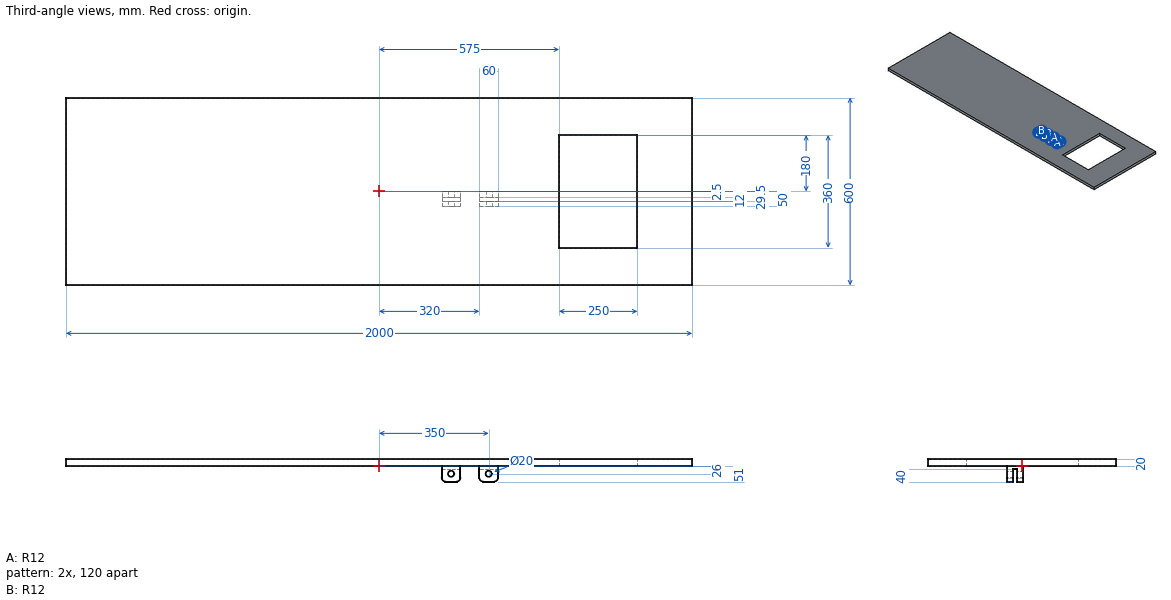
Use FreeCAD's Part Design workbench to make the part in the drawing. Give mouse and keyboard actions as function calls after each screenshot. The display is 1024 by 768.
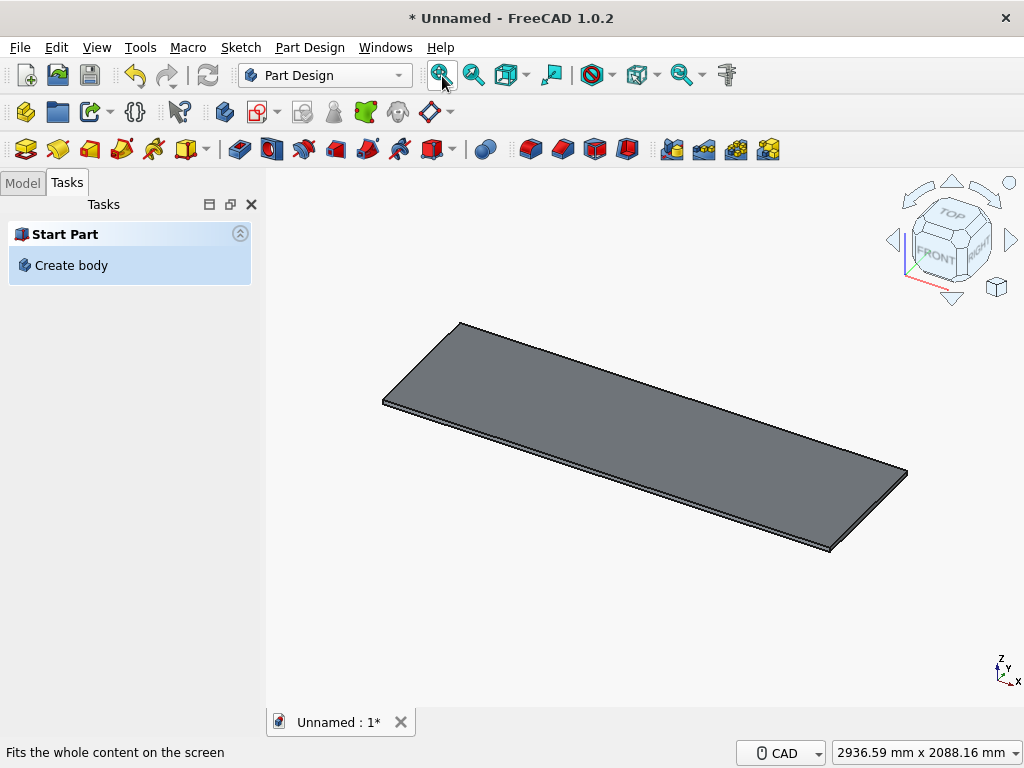
click(258, 112)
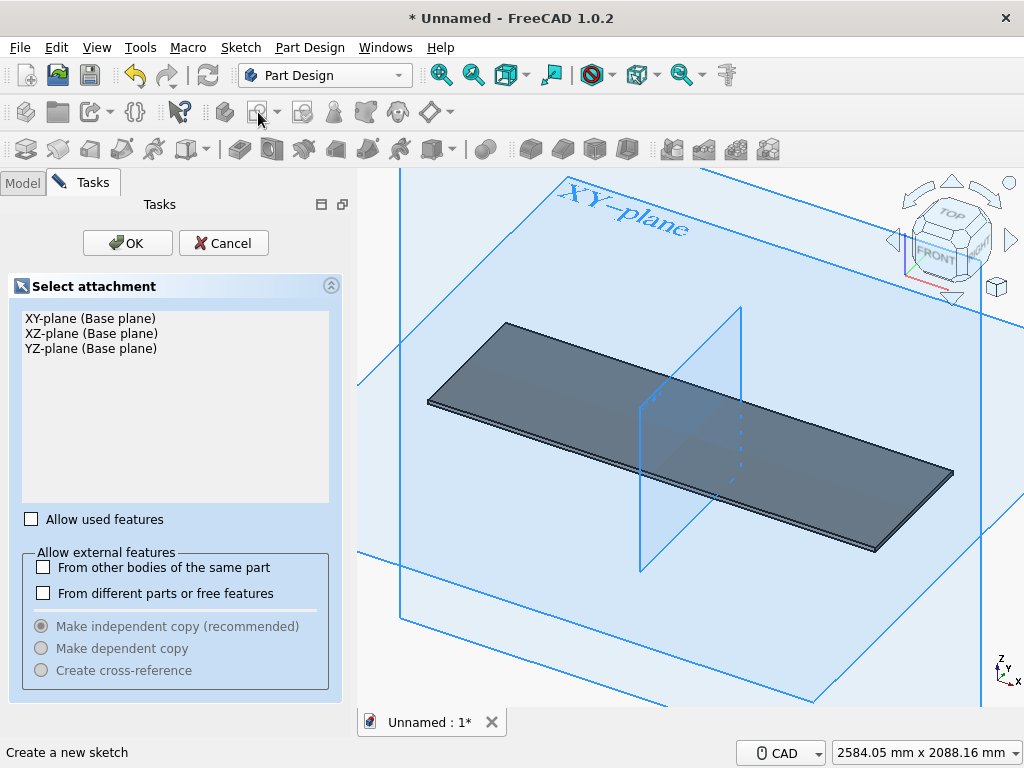
click(82, 318)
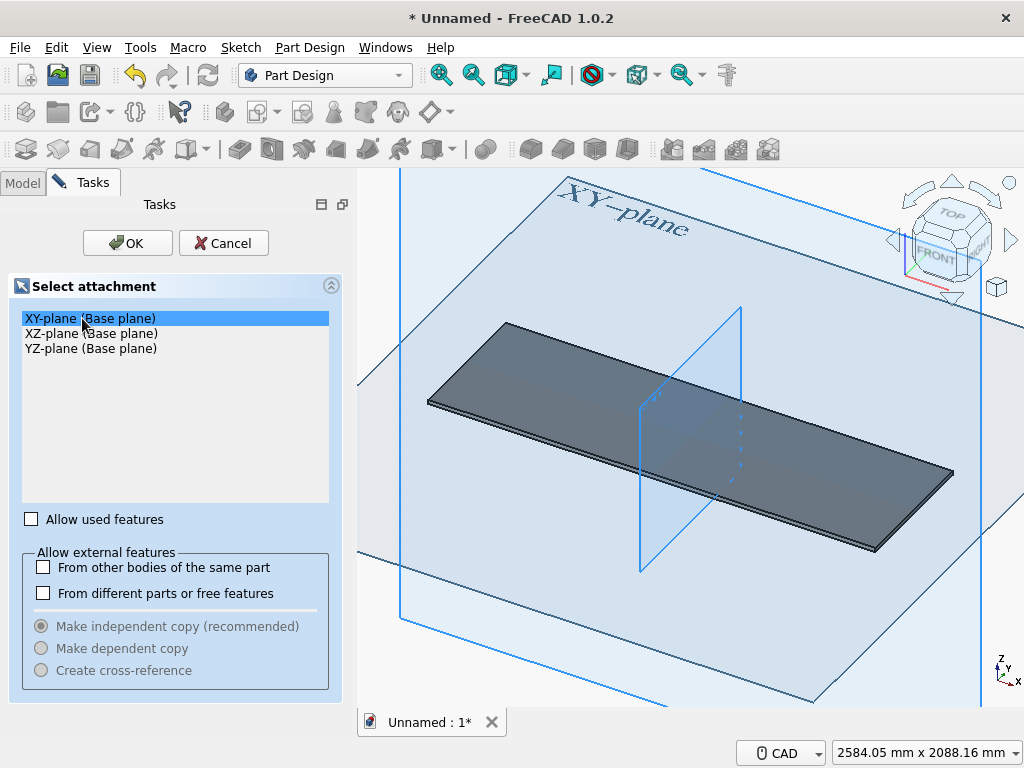
click(128, 243)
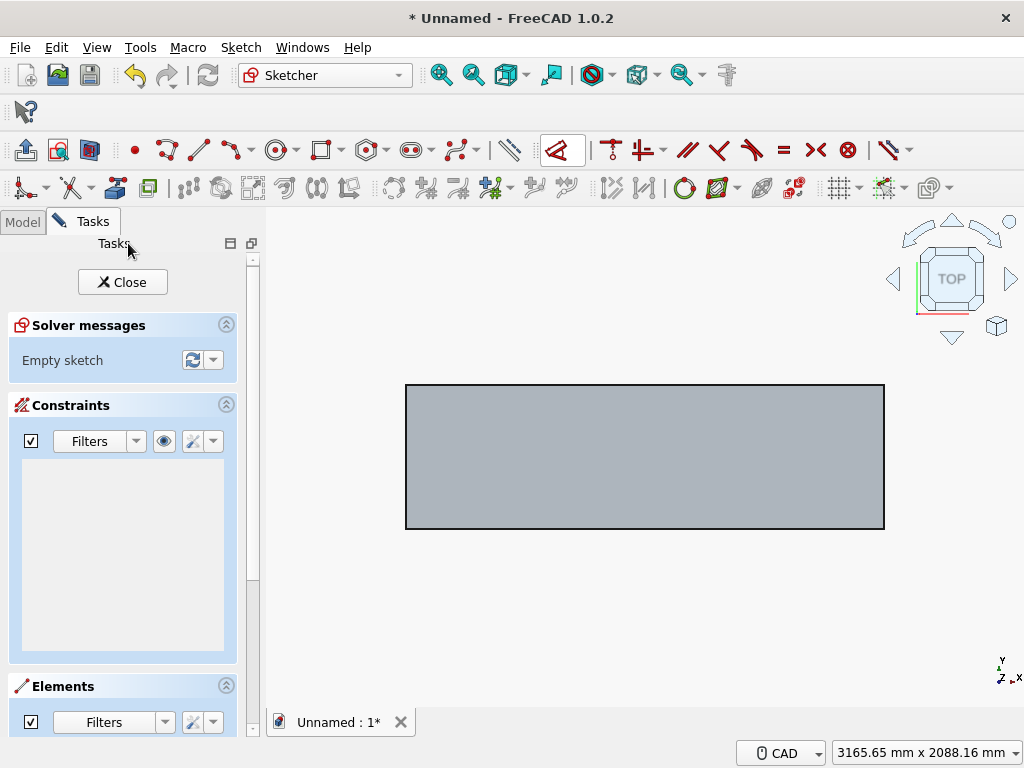
key(q)
key(s)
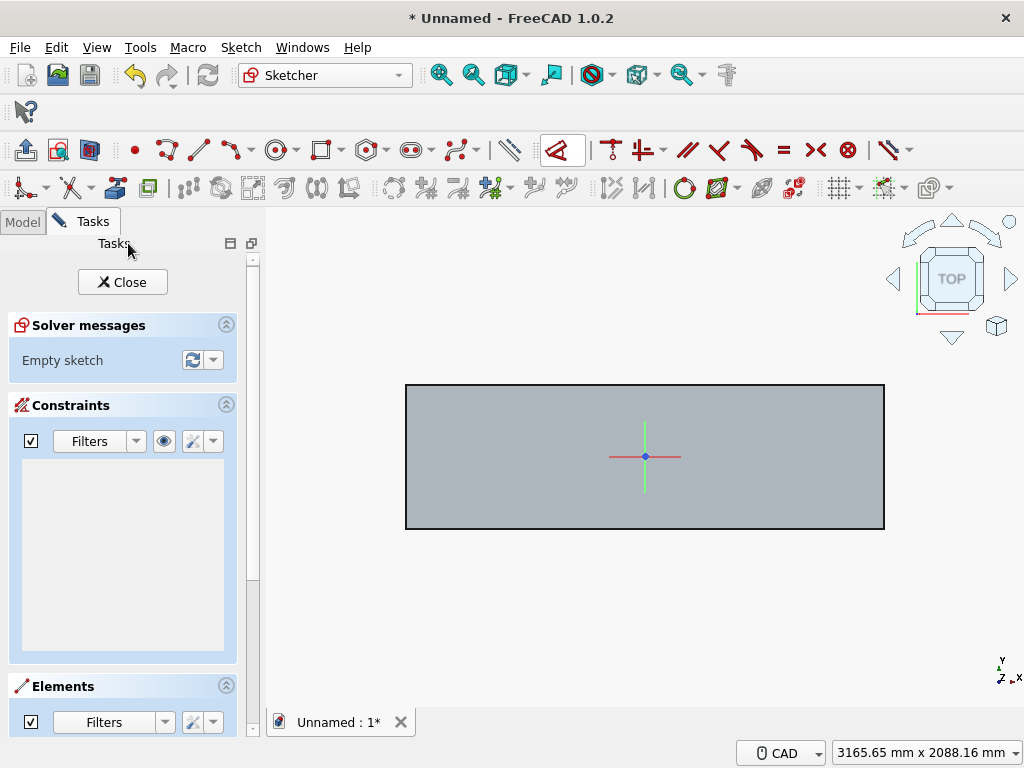
scroll(859, 457, up, 4)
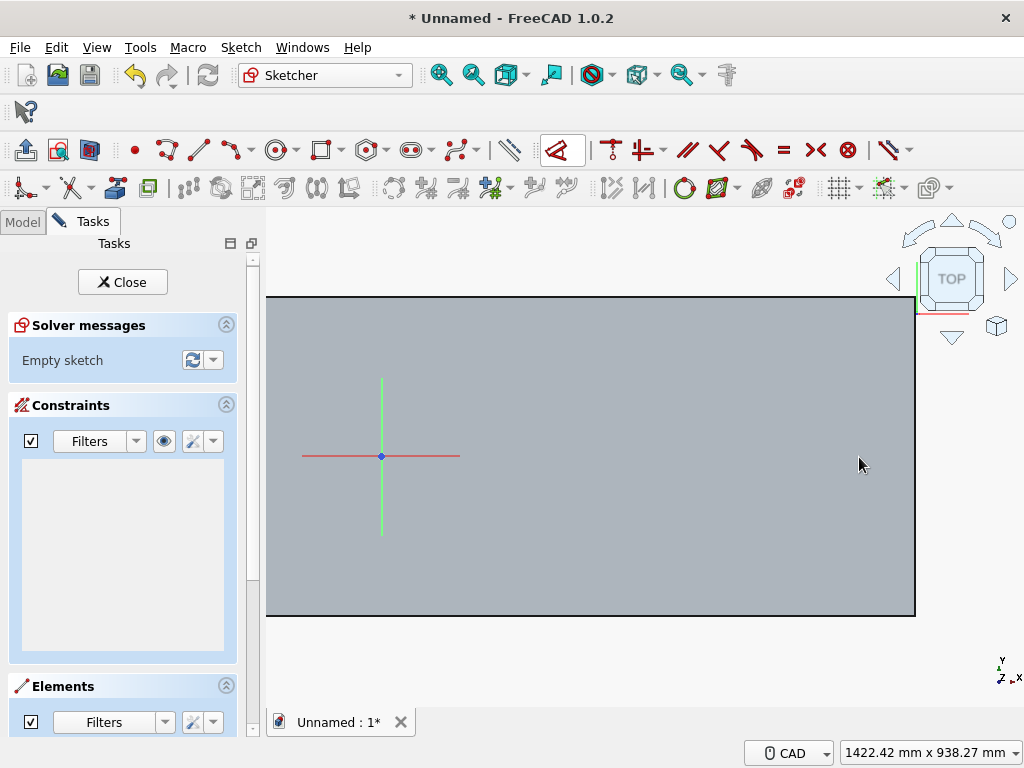
key(g)
key(r)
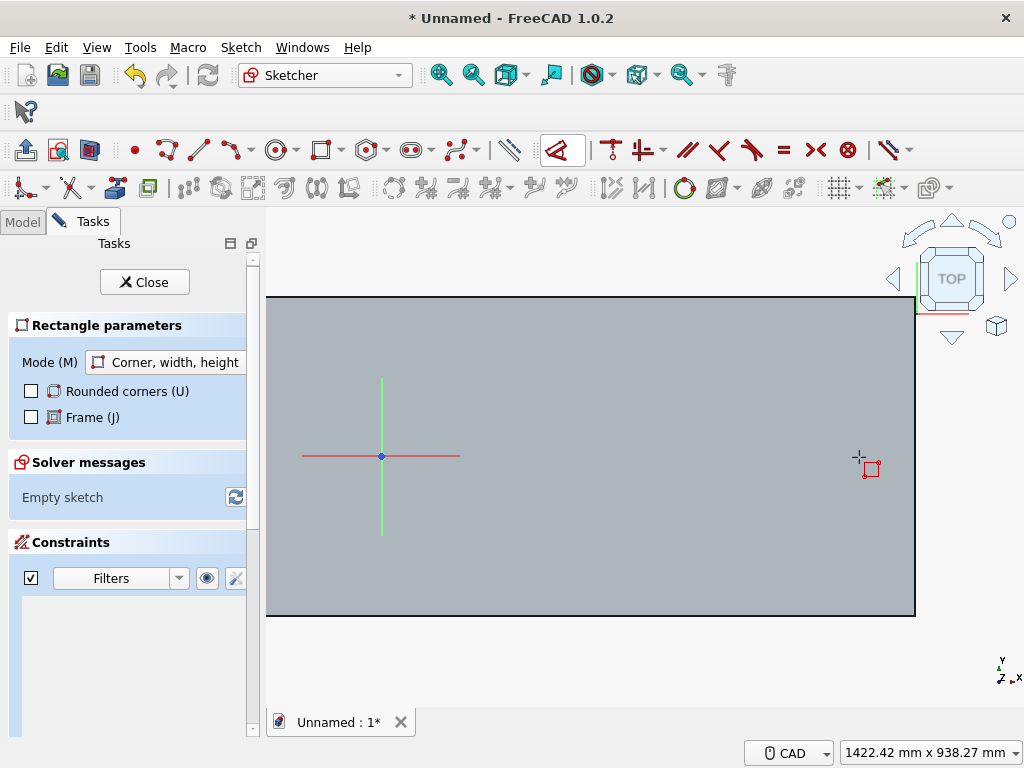
click(688, 360)
move(821, 552)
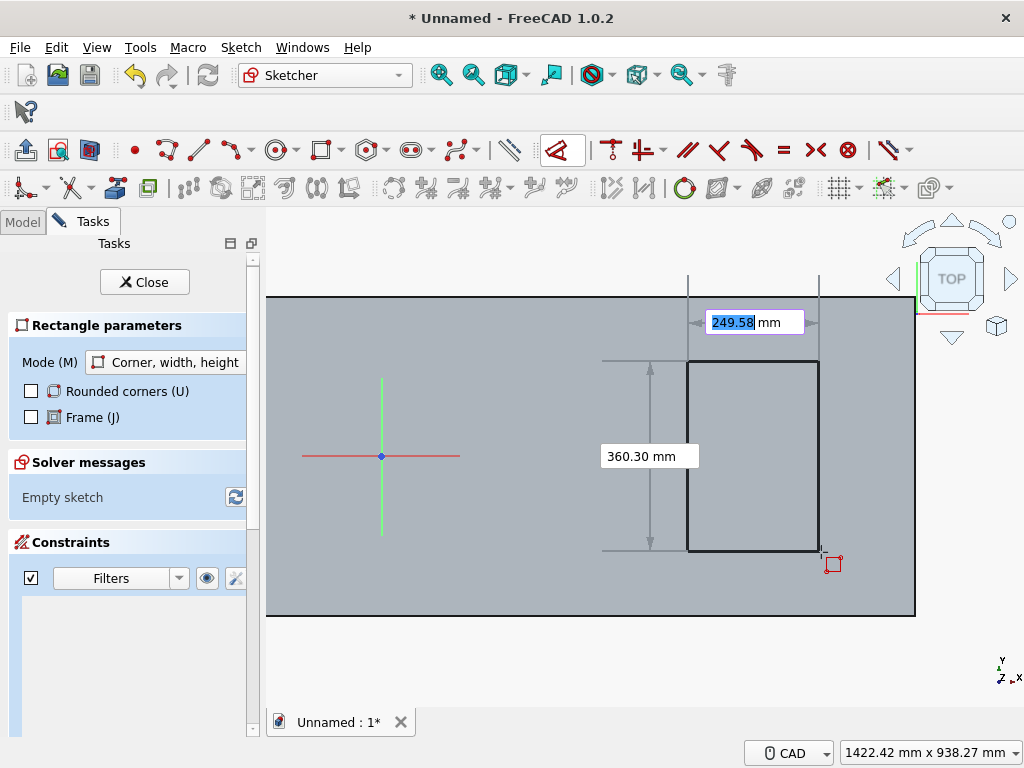
text(250)
key(Tab)
text(360)
key(Return)
key(Escape)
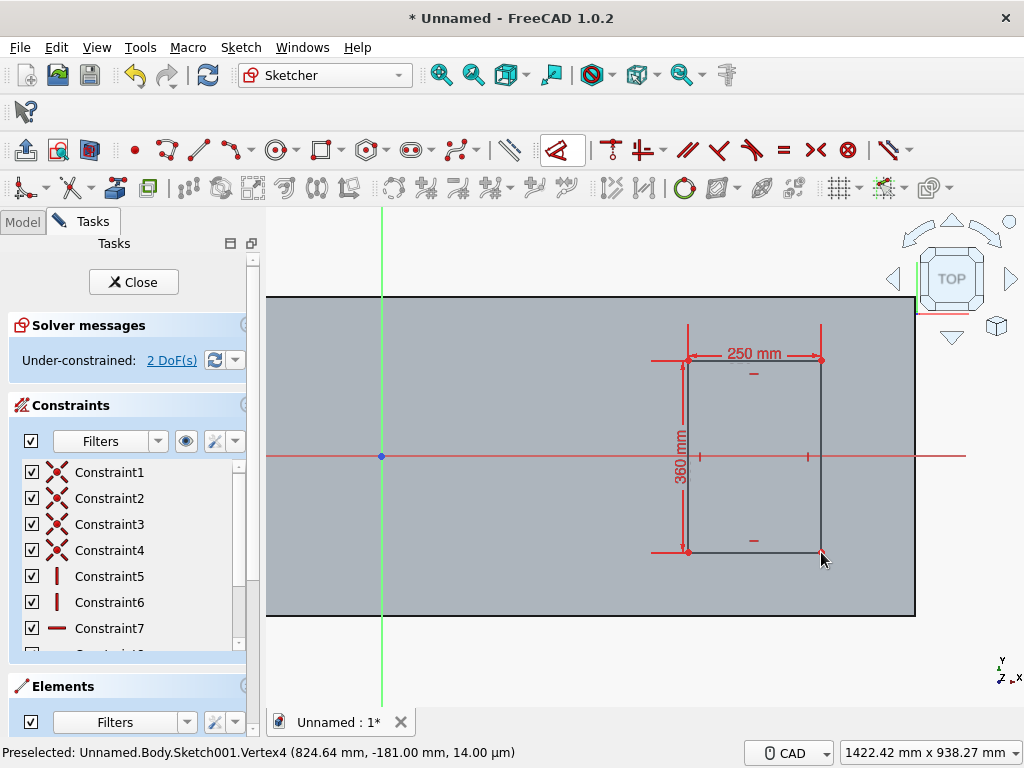
click(556, 150)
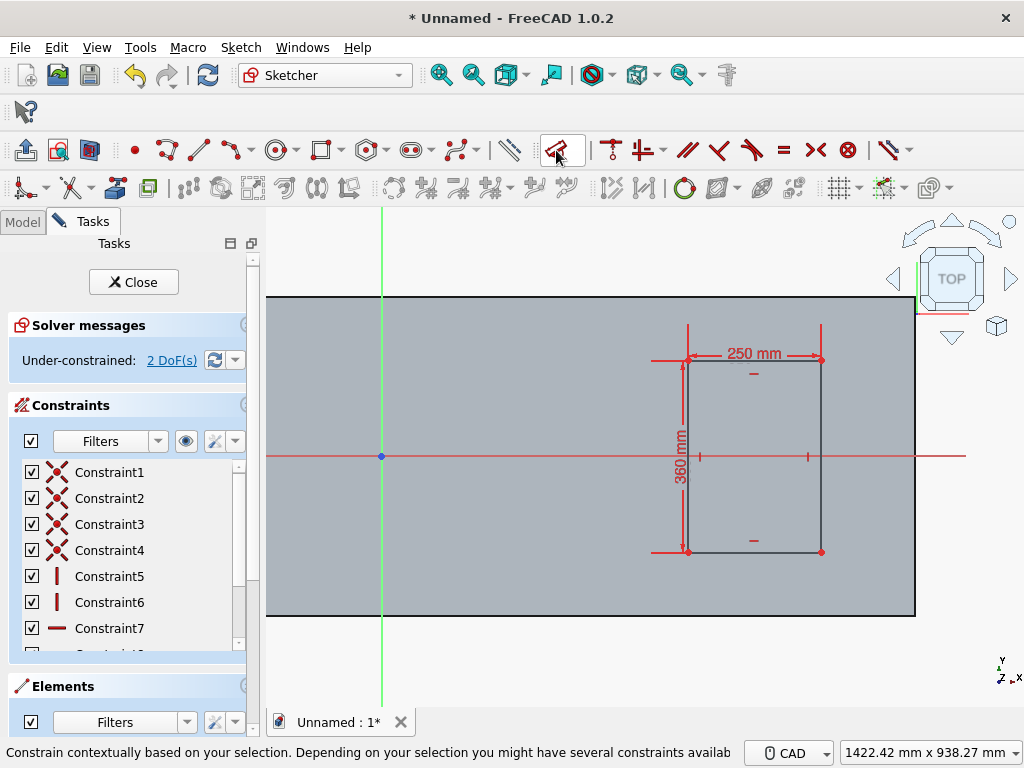
click(688, 361)
click(535, 327)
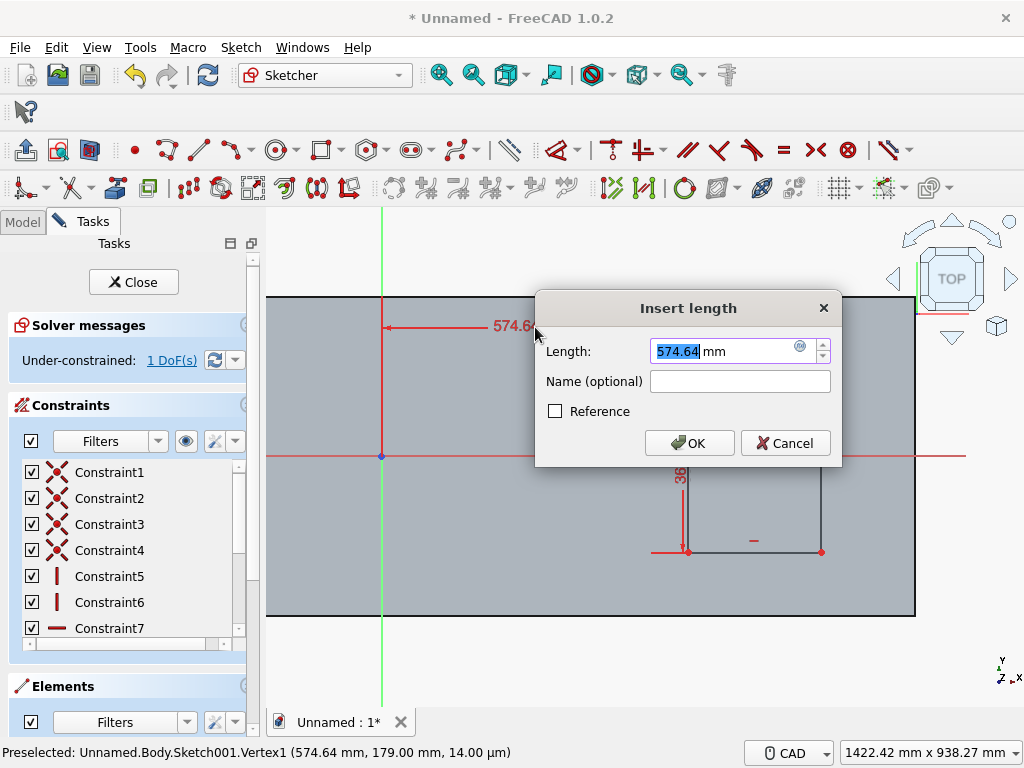
text(575)
key(Return)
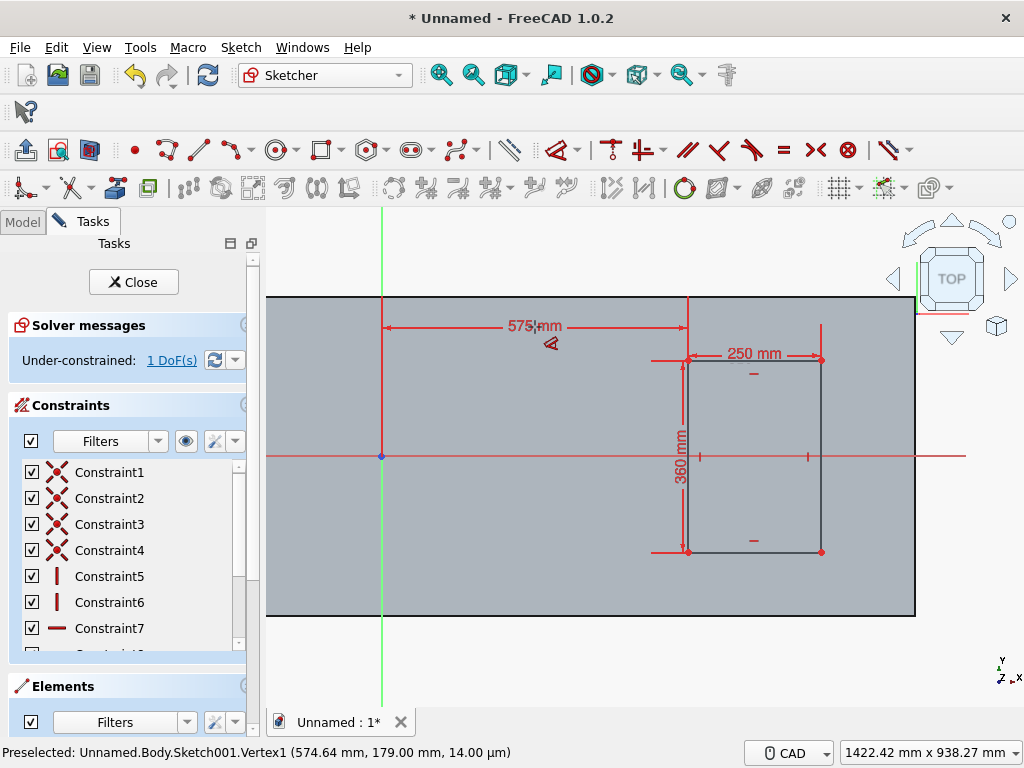
click(688, 361)
click(348, 409)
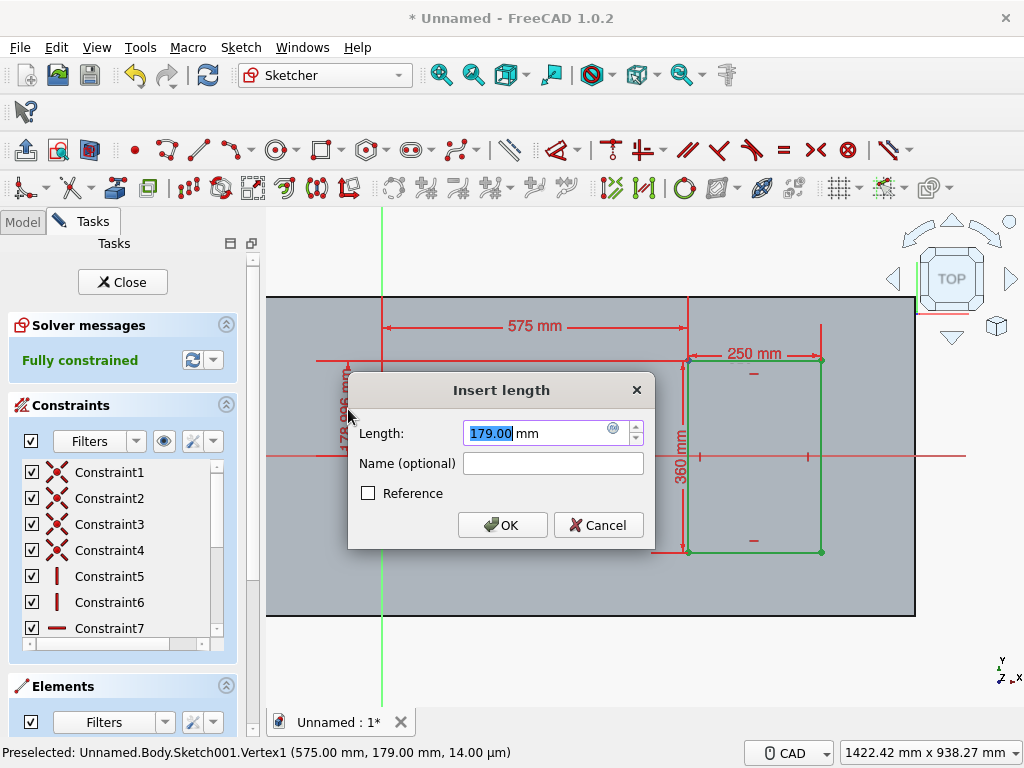
text(180)
key(Return)
key(Escape)